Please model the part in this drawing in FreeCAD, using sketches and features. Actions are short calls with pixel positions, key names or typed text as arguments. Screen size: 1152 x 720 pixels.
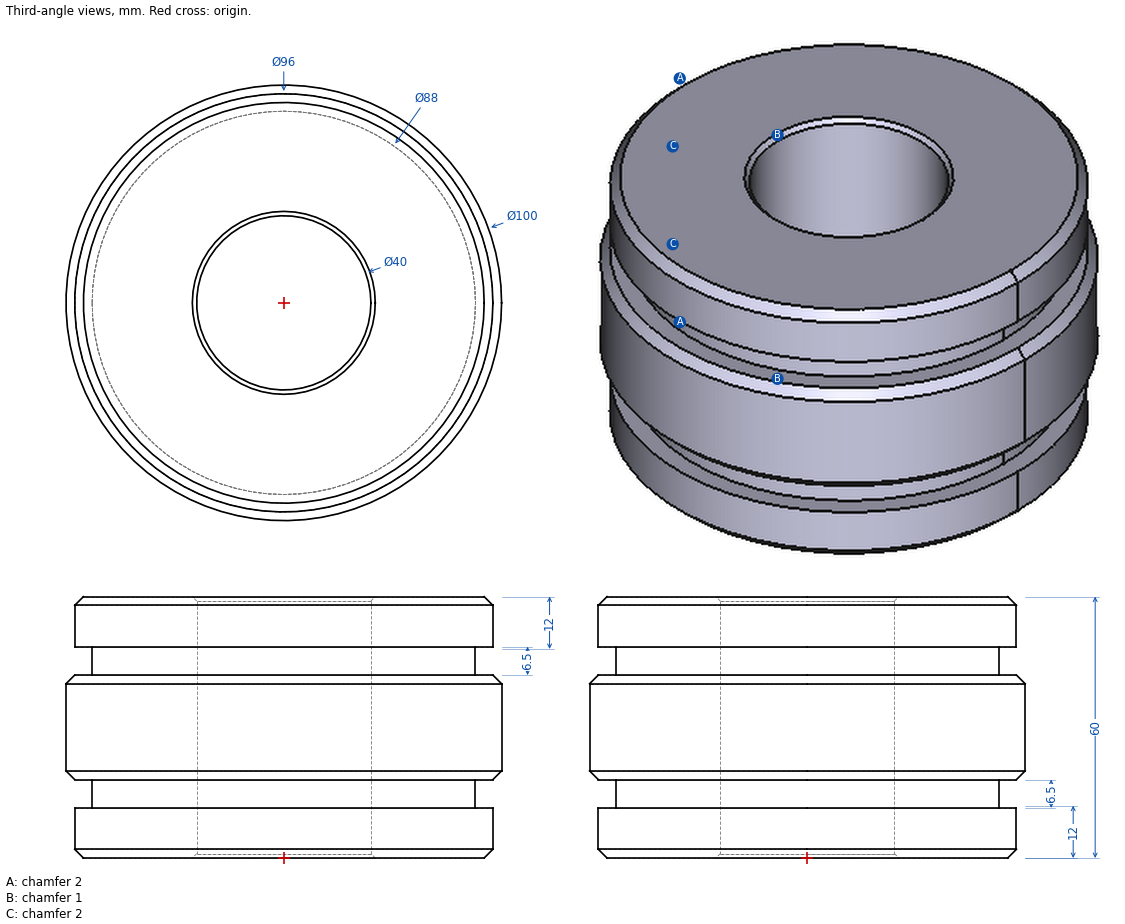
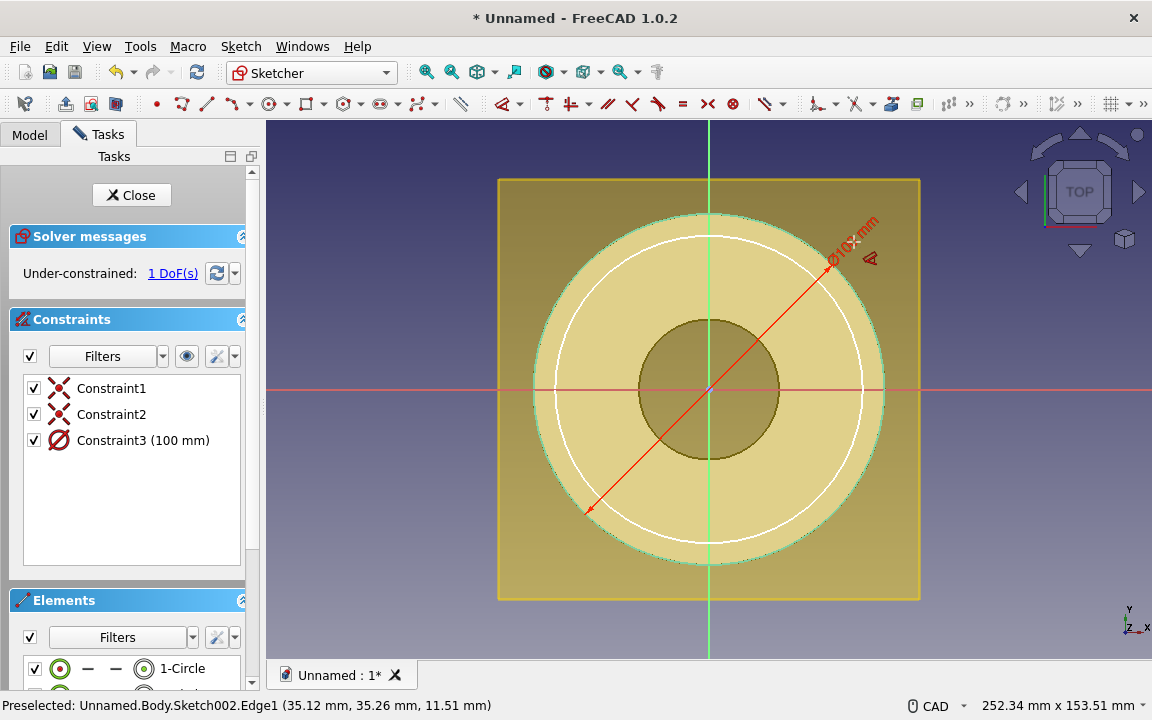
click(817, 280)
click(909, 329)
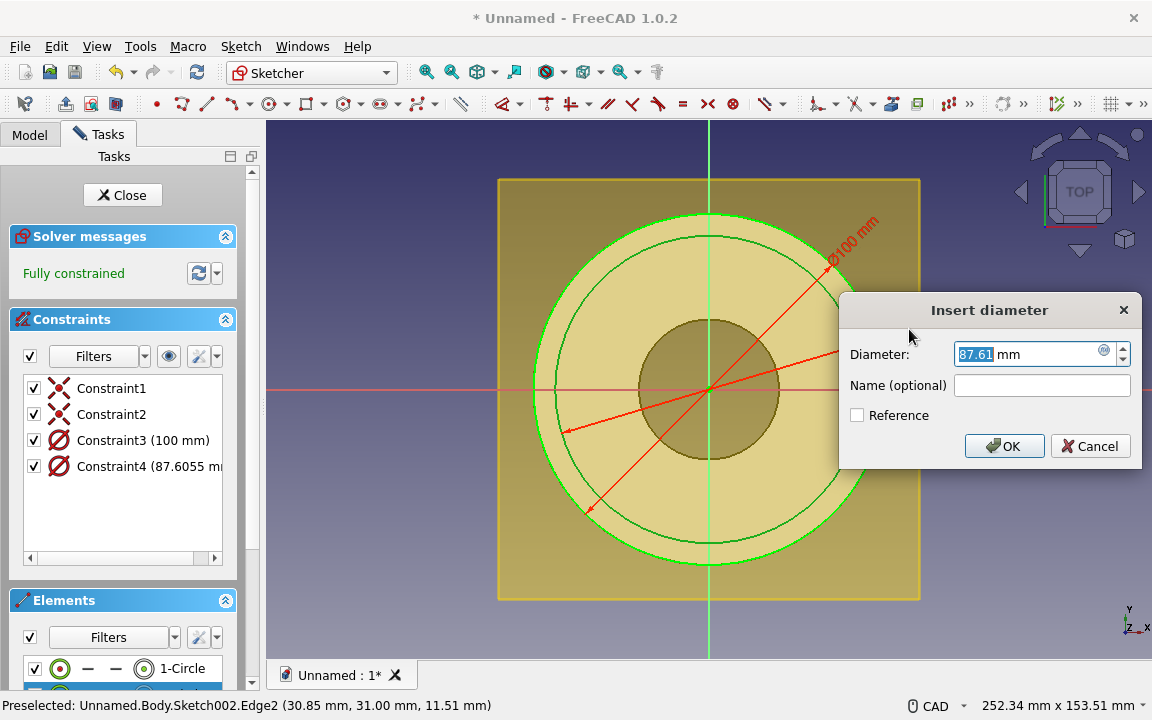
text(88)
key(Return)
key(Escape)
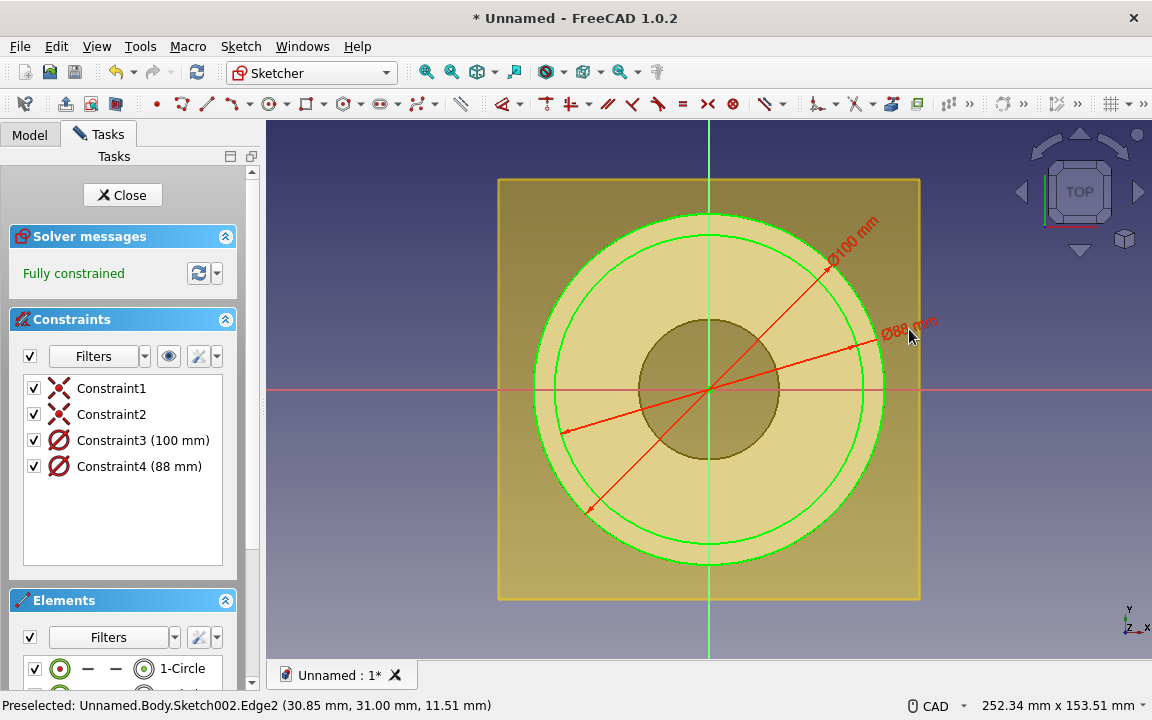
click(123, 195)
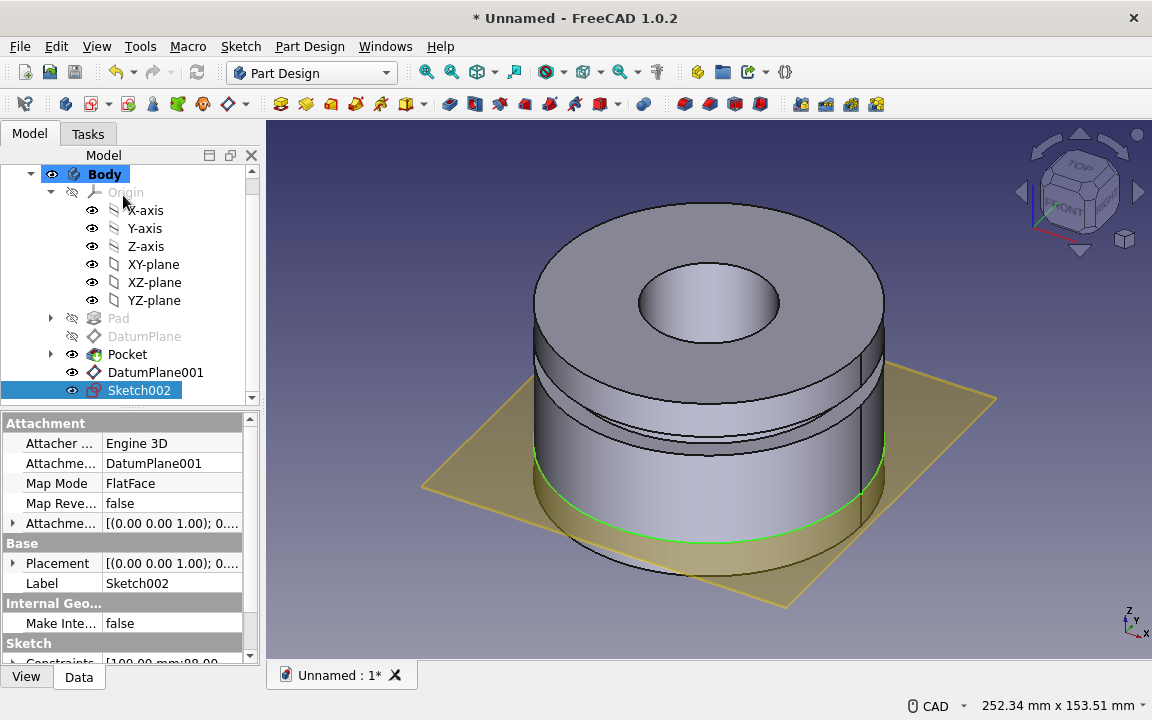
click(450, 104)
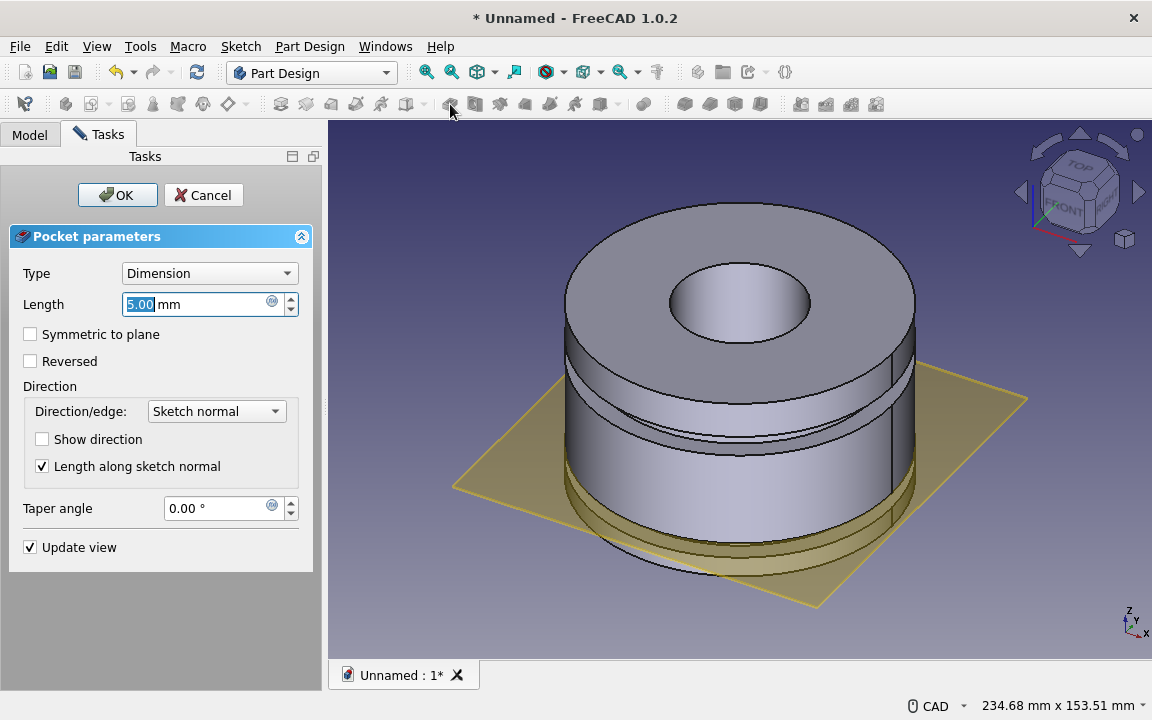
text(6.5)
key(Tab)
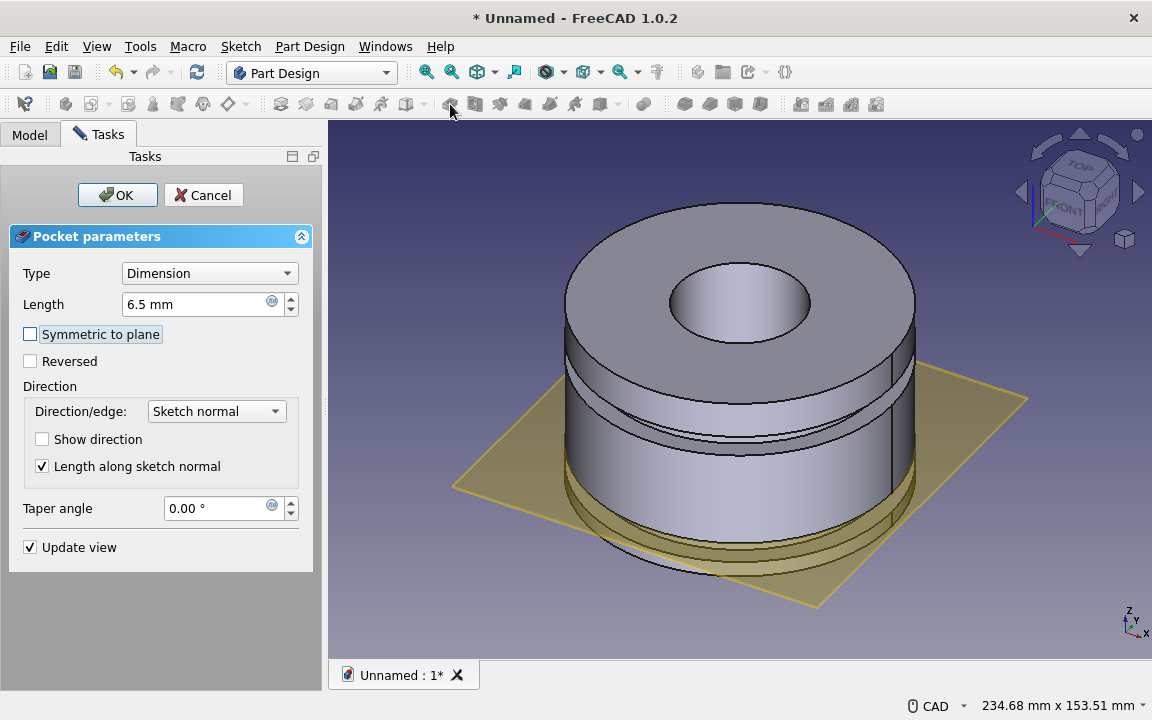
click(31, 361)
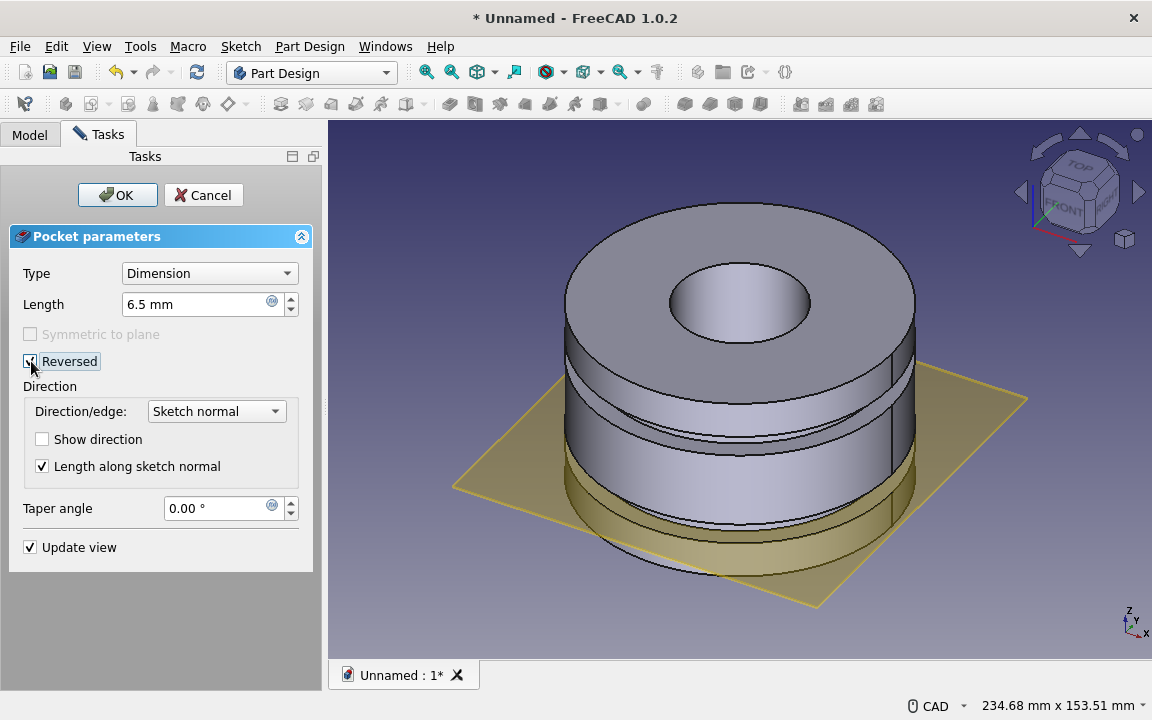
click(118, 195)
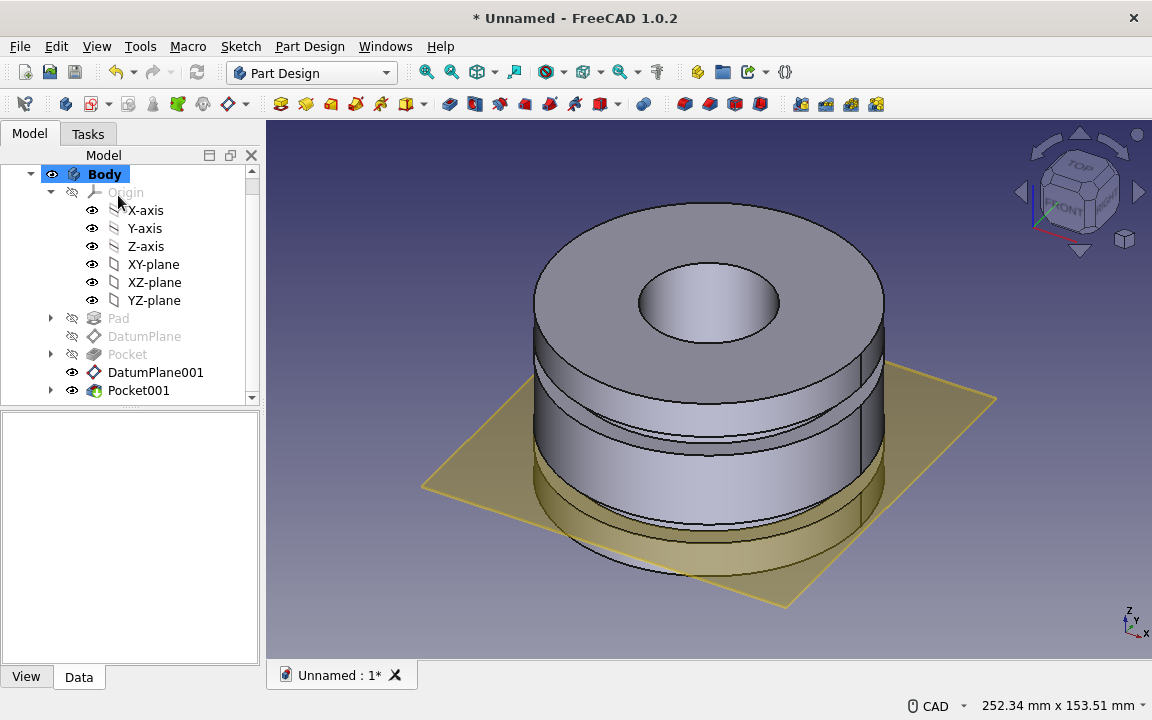
click(117, 372)
key(space)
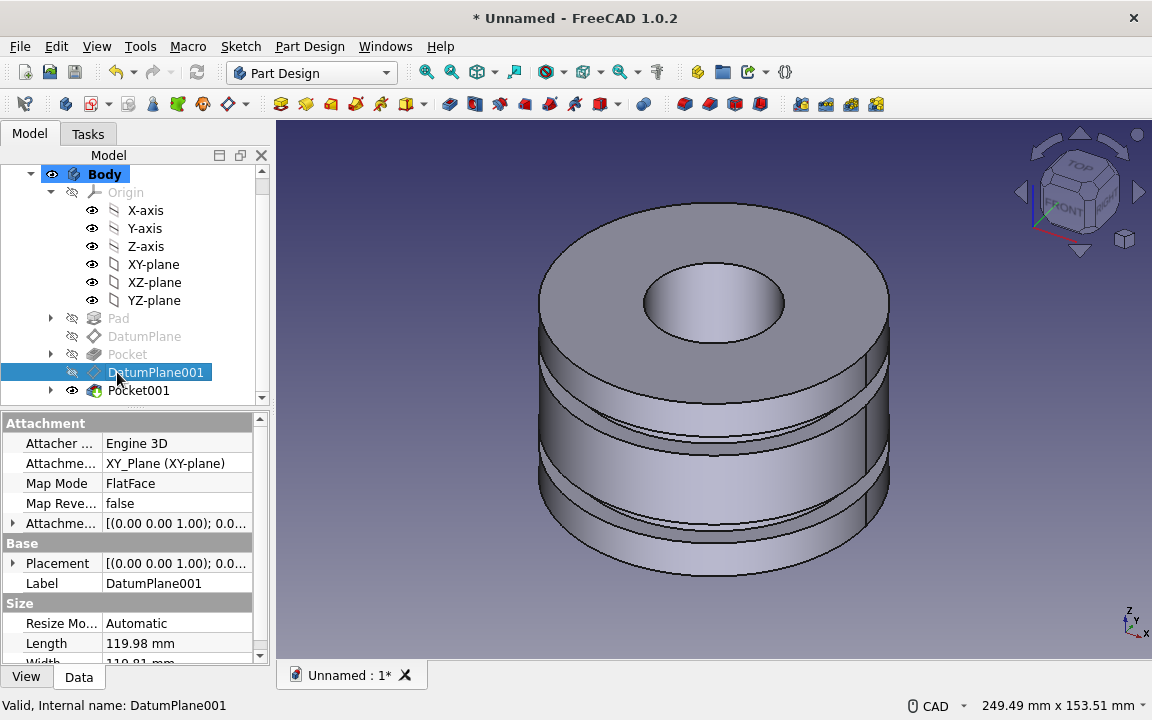
click(137, 264)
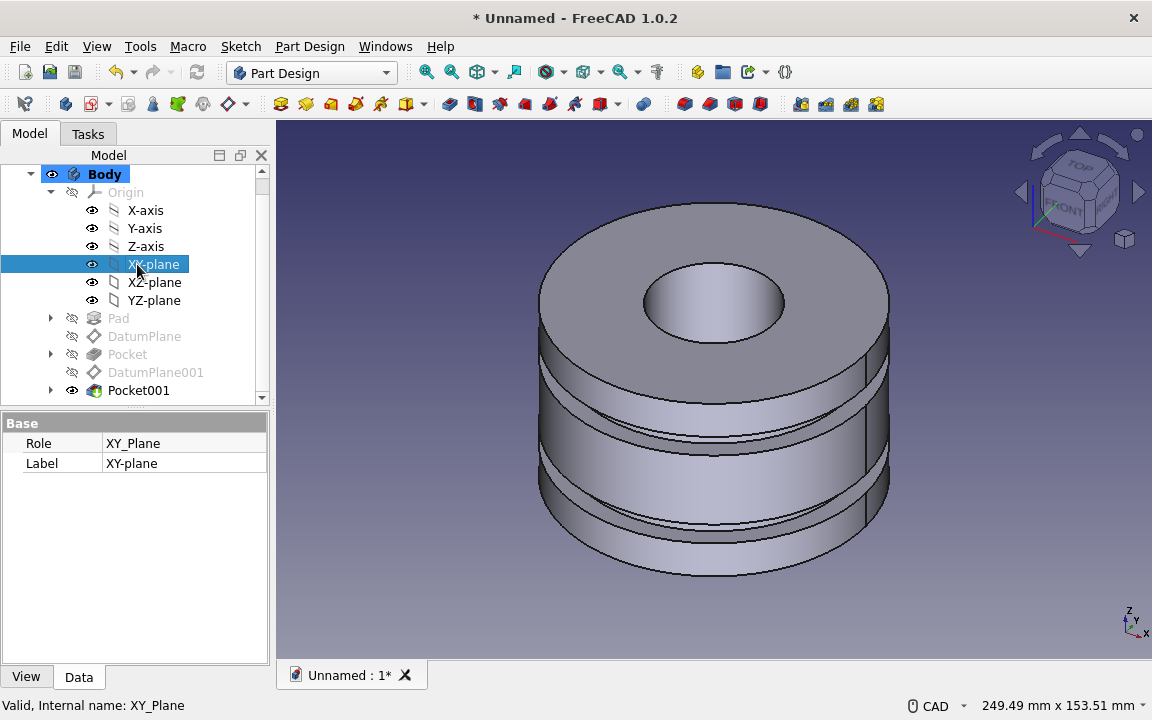
click(228, 104)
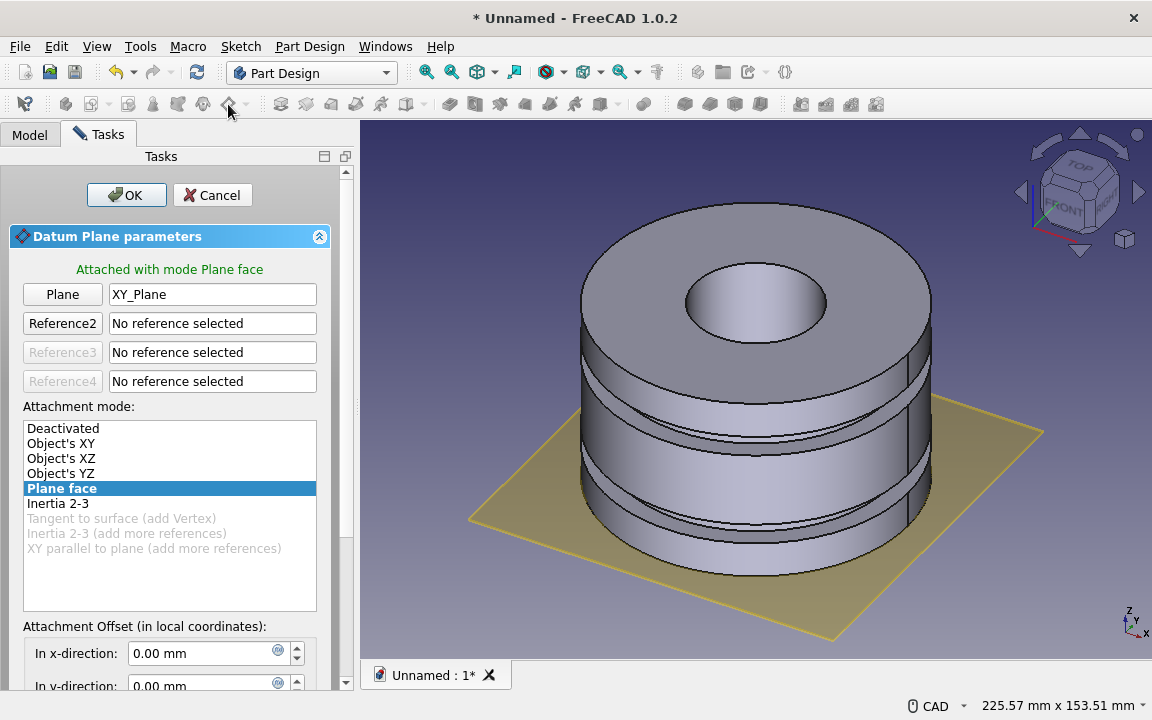
scroll(346, 428, down, 2)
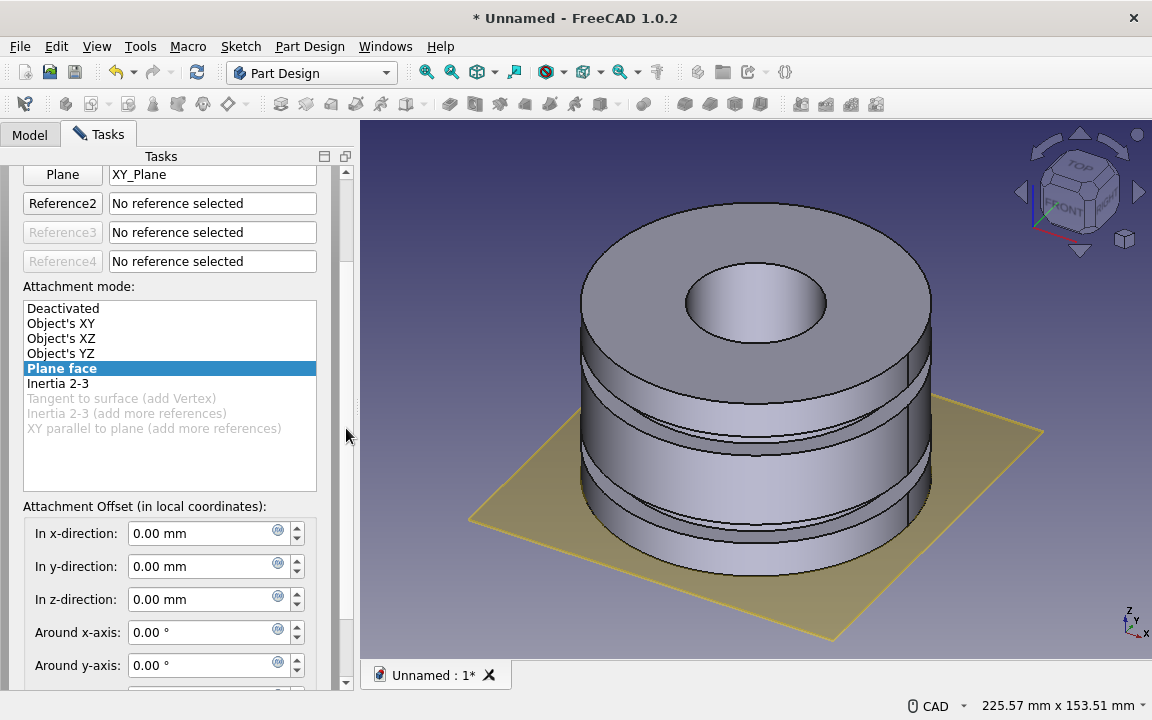
triple_click(210, 600)